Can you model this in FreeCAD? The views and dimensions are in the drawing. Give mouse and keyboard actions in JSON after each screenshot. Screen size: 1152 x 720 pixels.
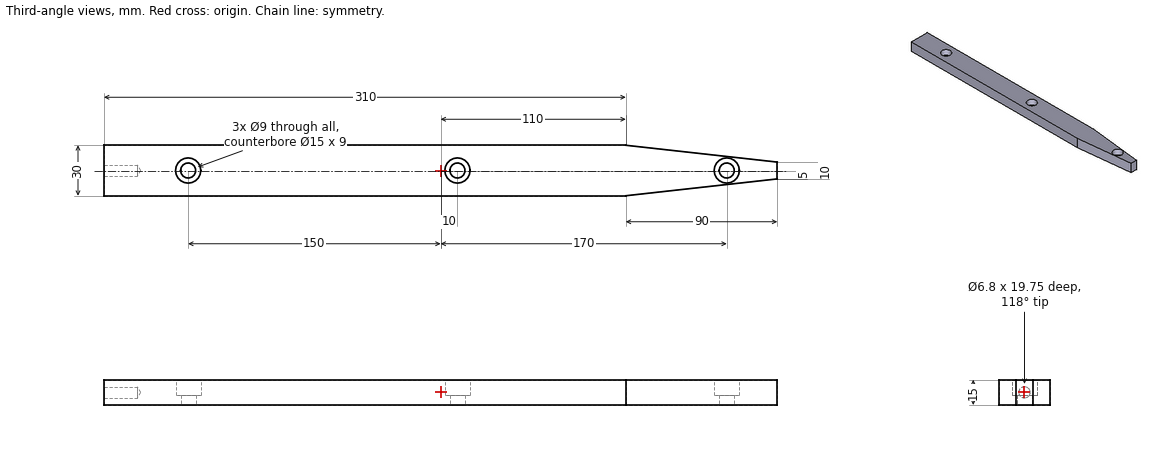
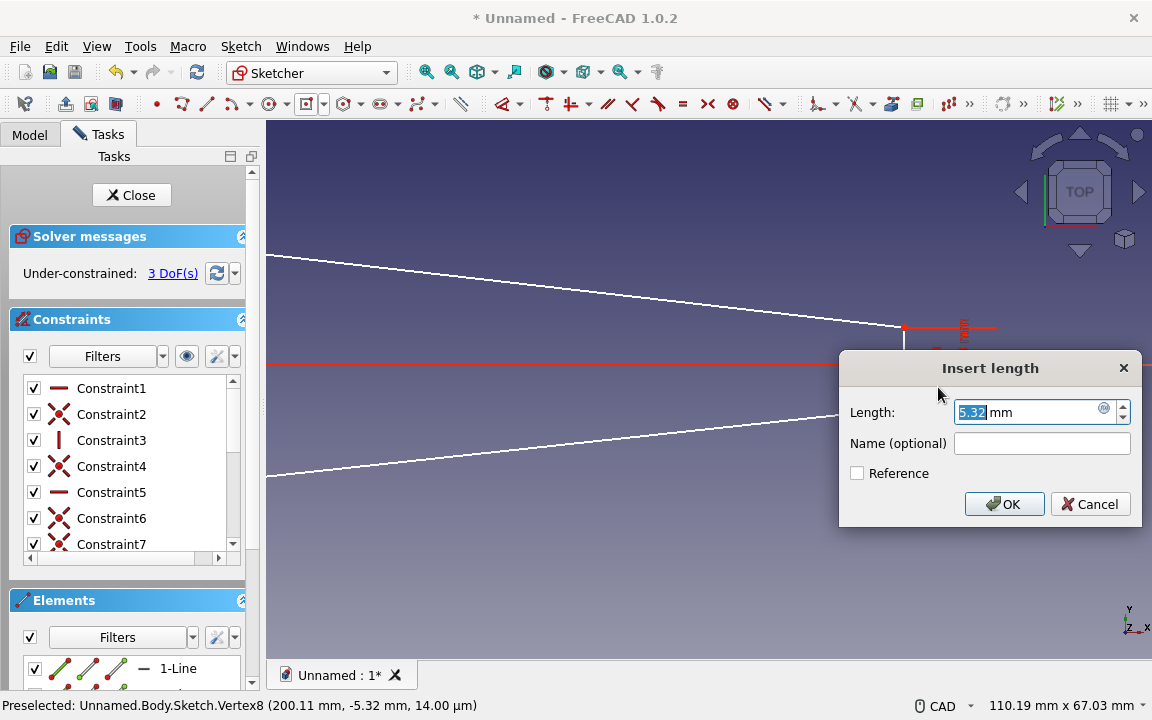
{"action": "type", "text": "5"}
{"action": "key", "text": "Return"}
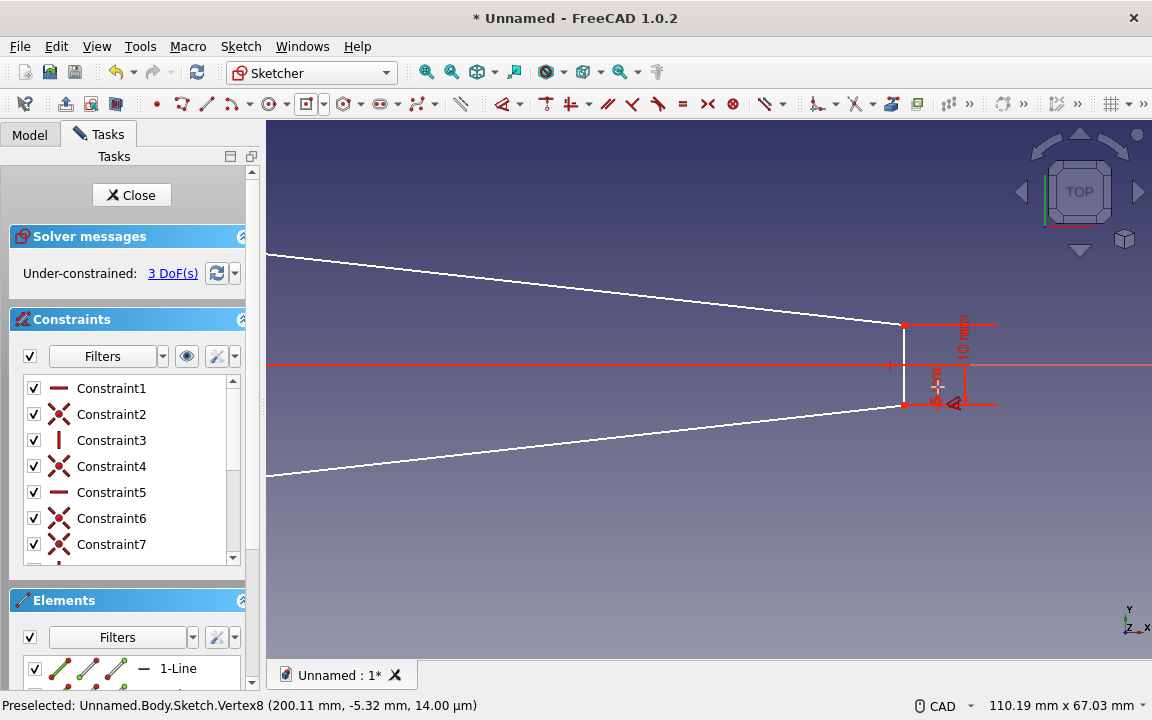
{"action": "scroll", "coordinate": [907, 394], "scroll_direction": "down", "scroll_amount": 9}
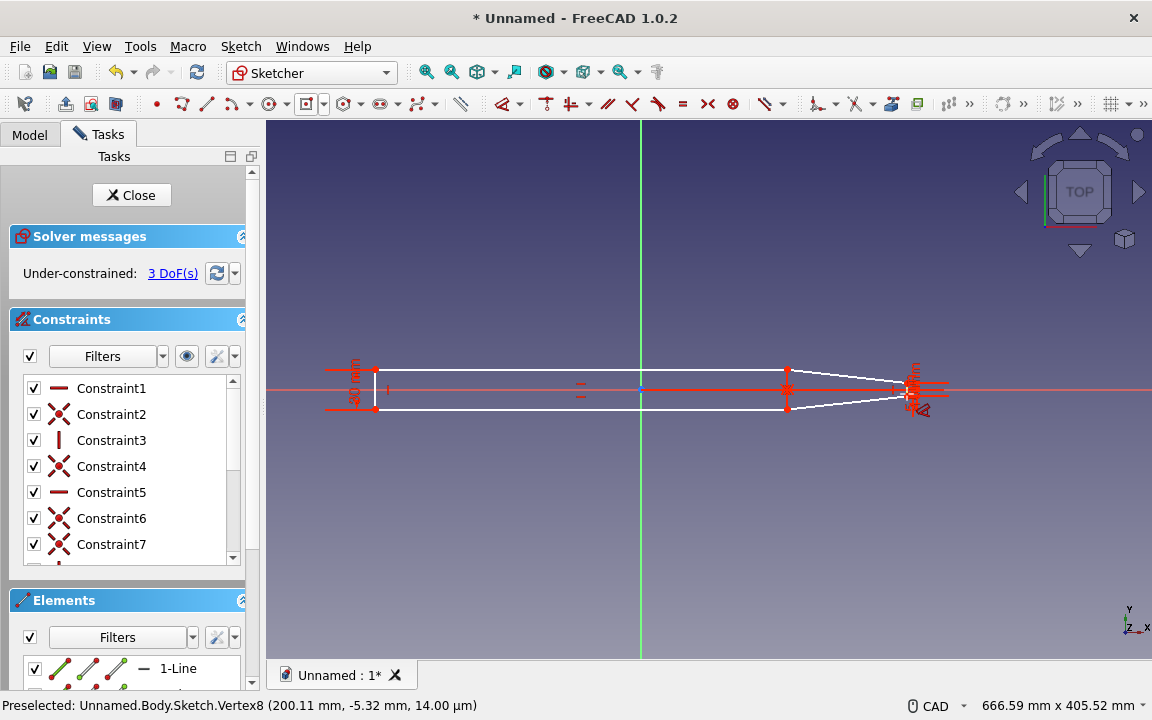
{"action": "left_click", "coordinate": [664, 370]}
{"action": "left_click", "coordinate": [581, 336]}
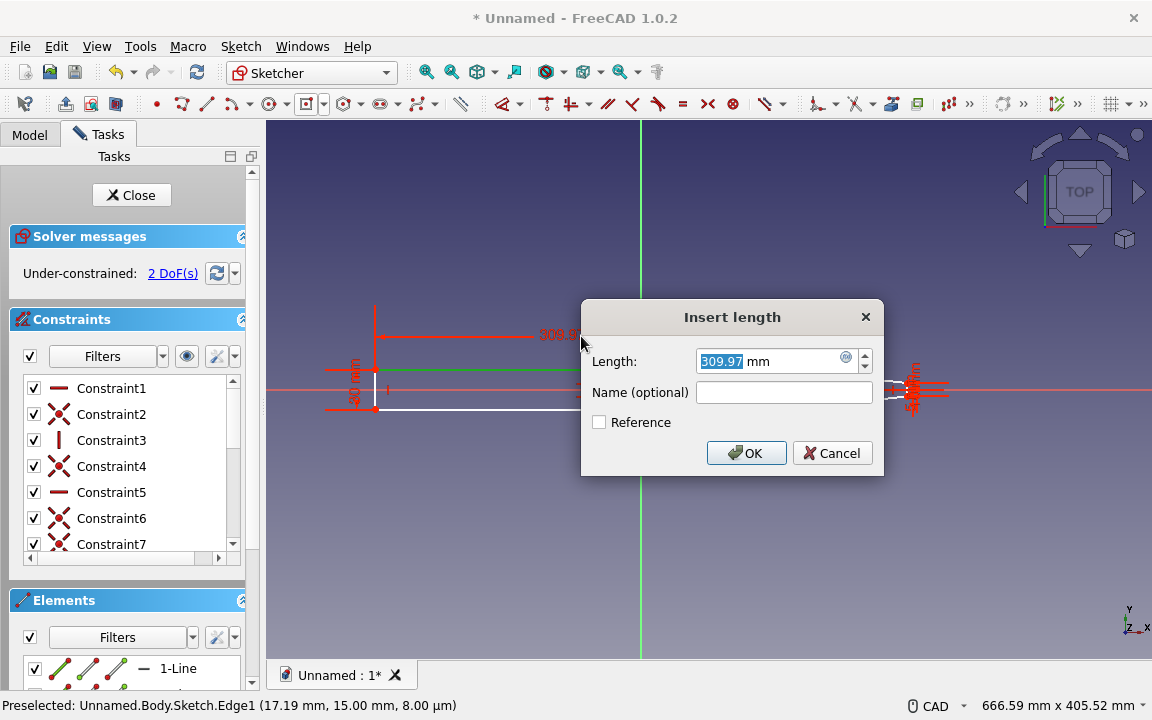
{"action": "type", "text": "310"}
{"action": "key", "text": "Return"}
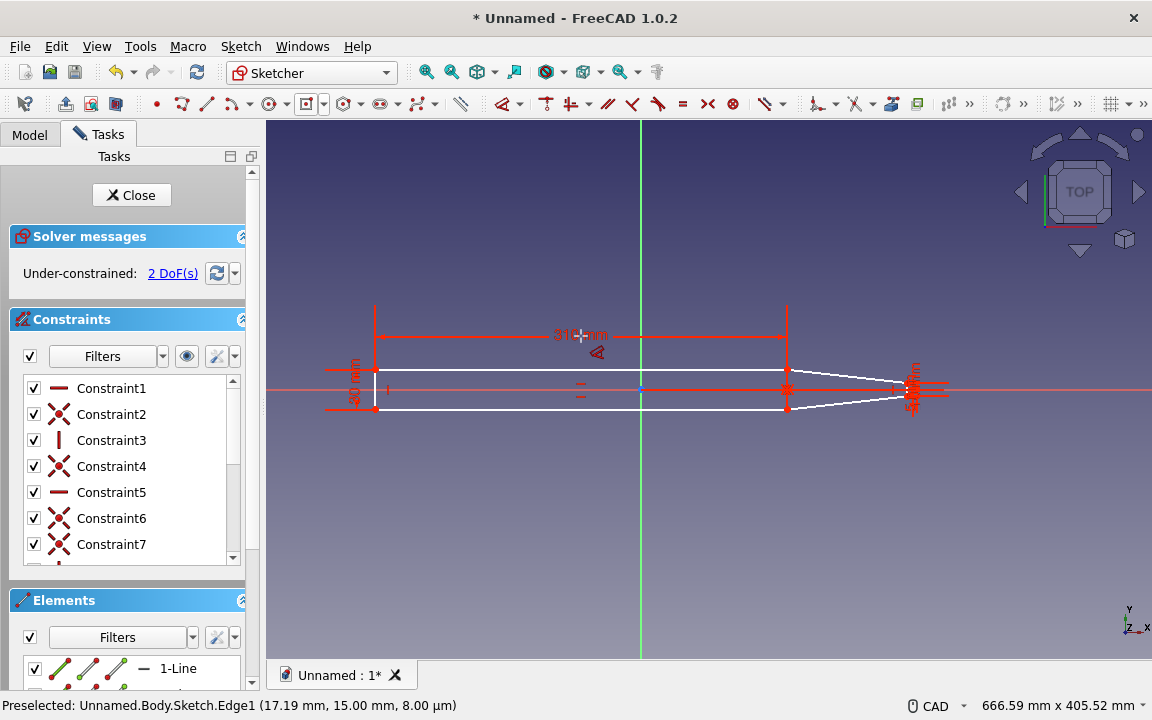
{"action": "left_click", "coordinate": [823, 406]}
{"action": "left_click", "coordinate": [847, 444]}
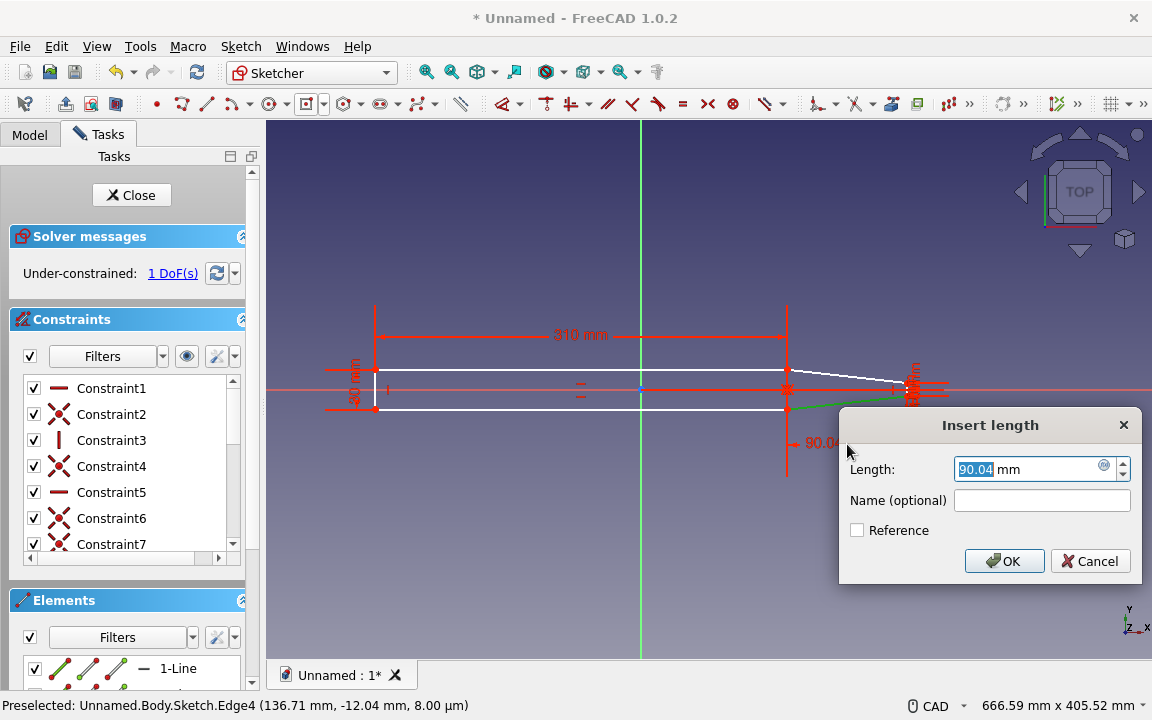
{"action": "type", "text": "90"}
{"action": "key", "text": "Return"}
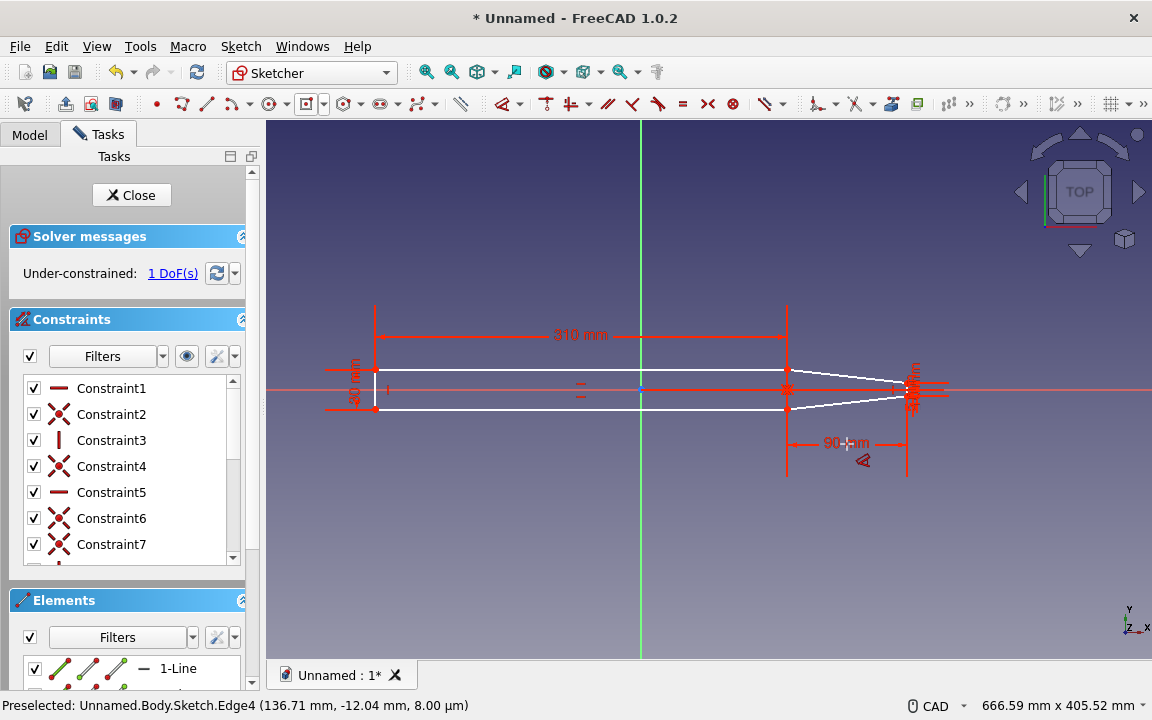
{"action": "left_click", "coordinate": [787, 370]}
{"action": "left_click", "coordinate": [714, 336]}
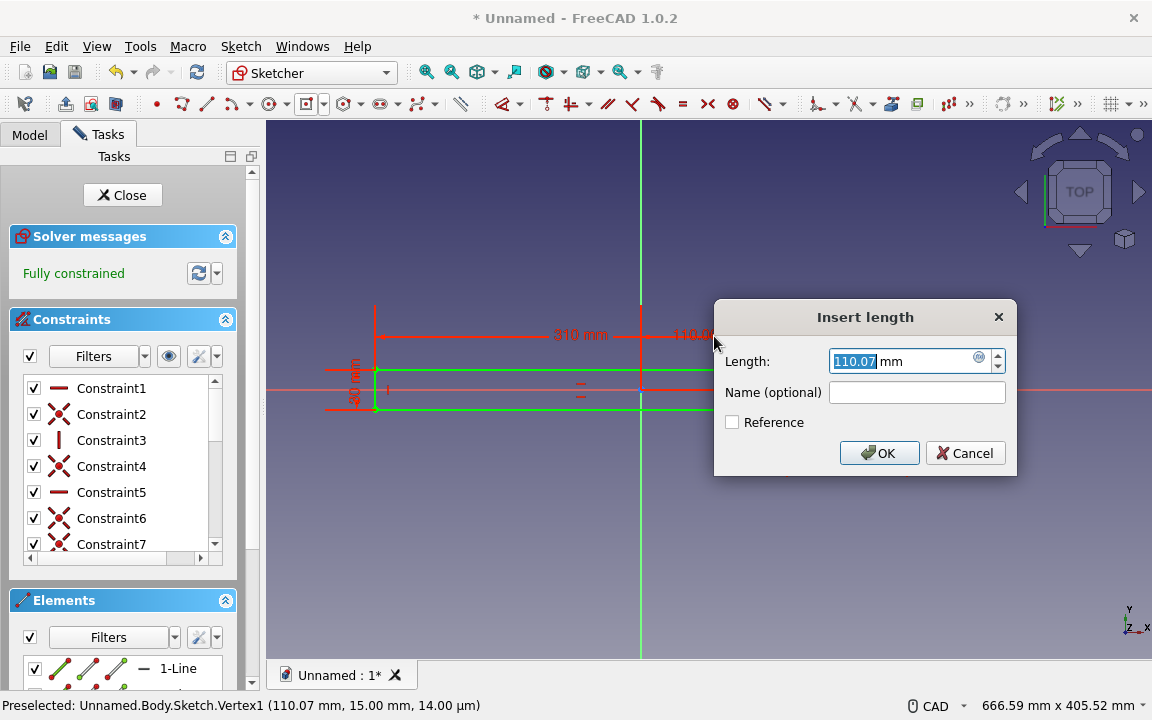
{"action": "type", "text": "110"}
{"action": "key", "text": "Return"}
{"action": "key", "text": "Escape"}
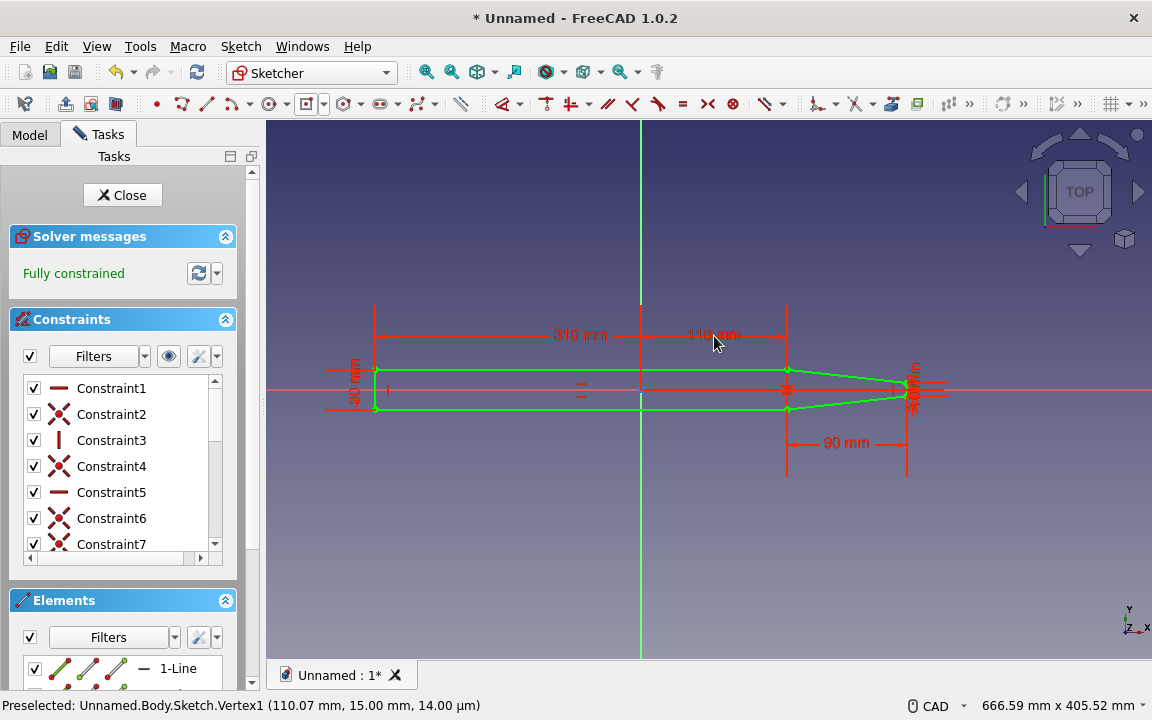
{"action": "left_click", "coordinate": [123, 195]}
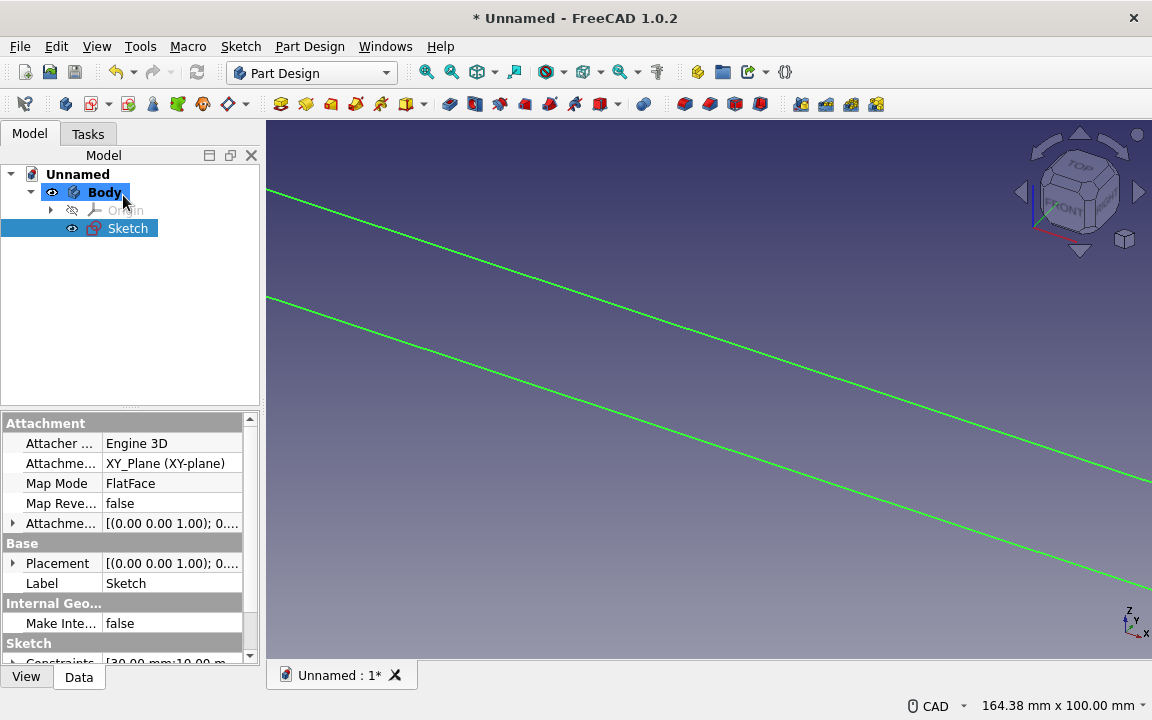
{"action": "left_click", "coordinate": [281, 104]}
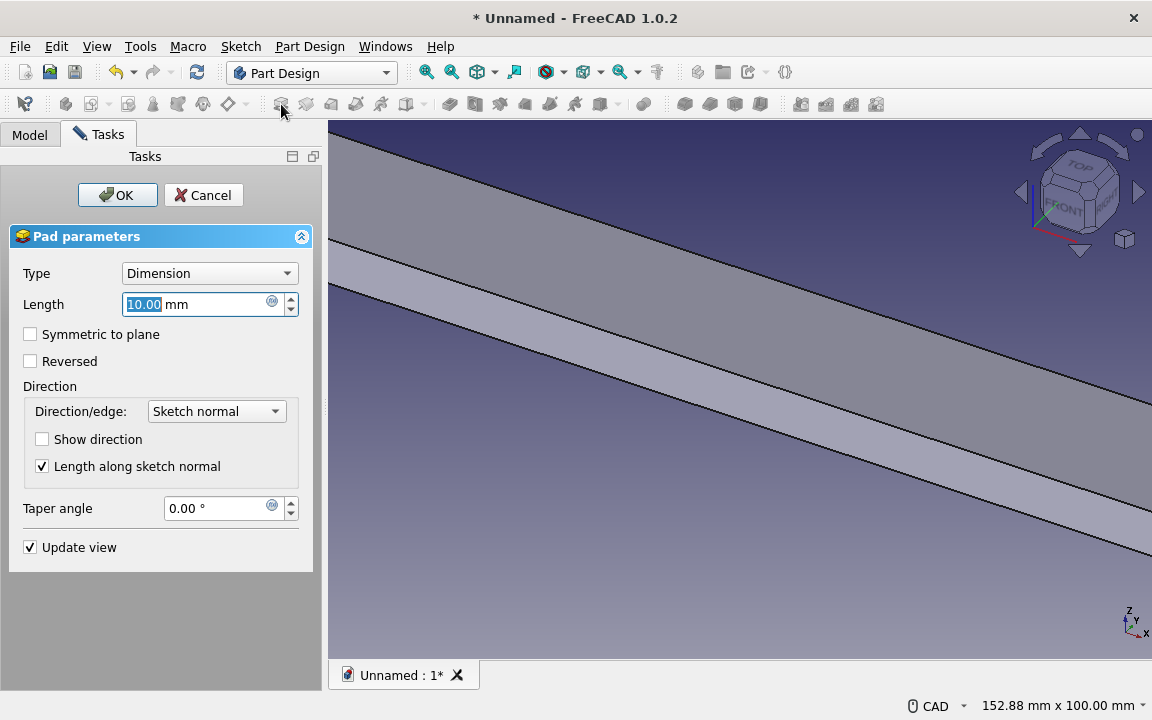
{"action": "type", "text": "15"}
{"action": "key", "text": "Tab"}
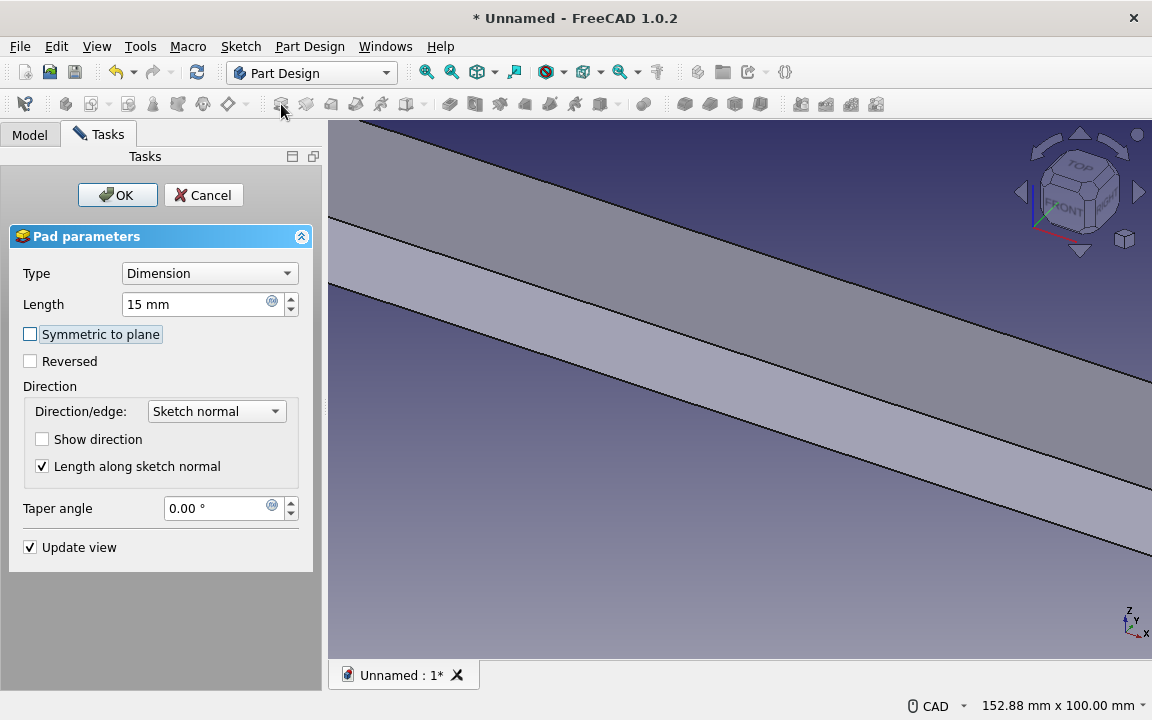
{"action": "left_click", "coordinate": [31, 334]}